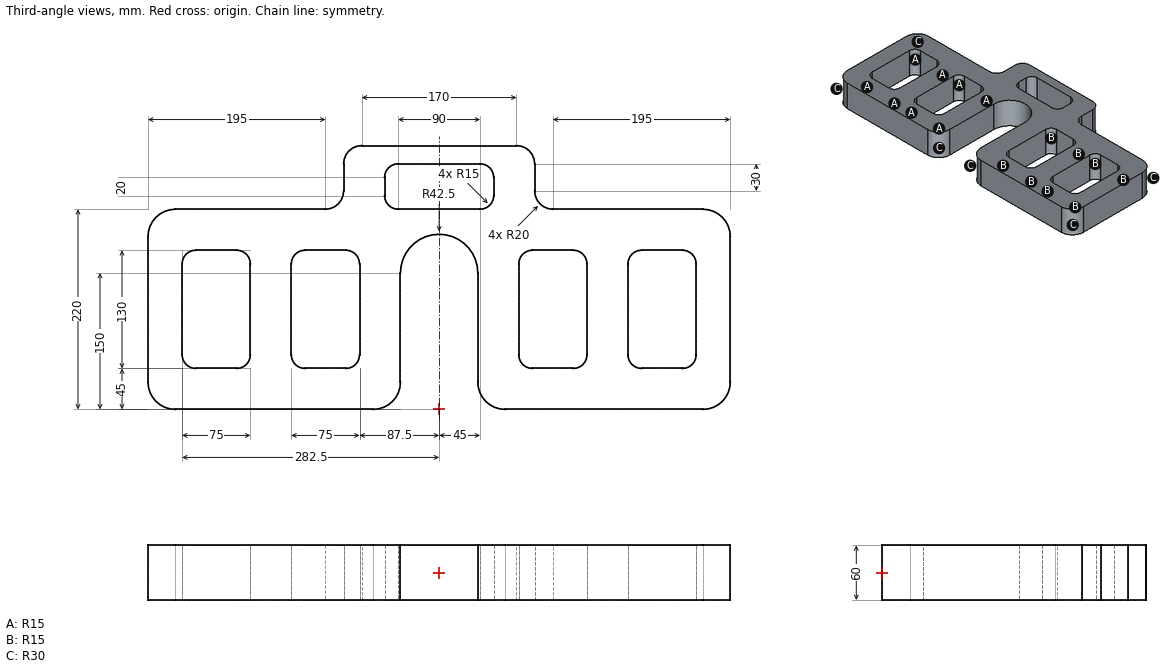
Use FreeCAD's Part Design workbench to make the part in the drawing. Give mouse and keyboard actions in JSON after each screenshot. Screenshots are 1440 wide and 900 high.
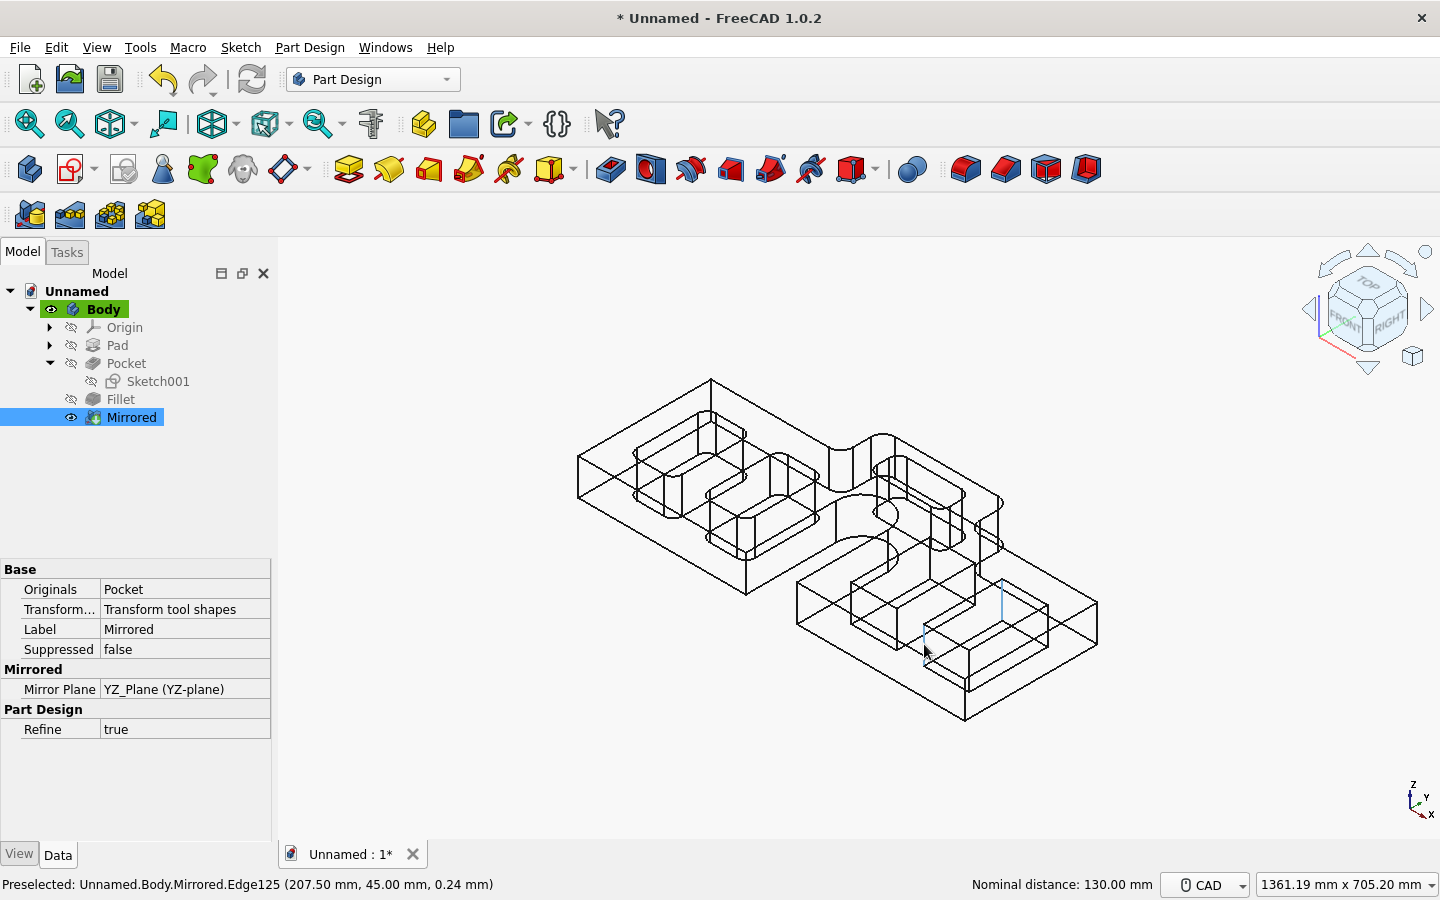
{"action": "left_click", "coordinate": [969, 666], "text": "ctrl"}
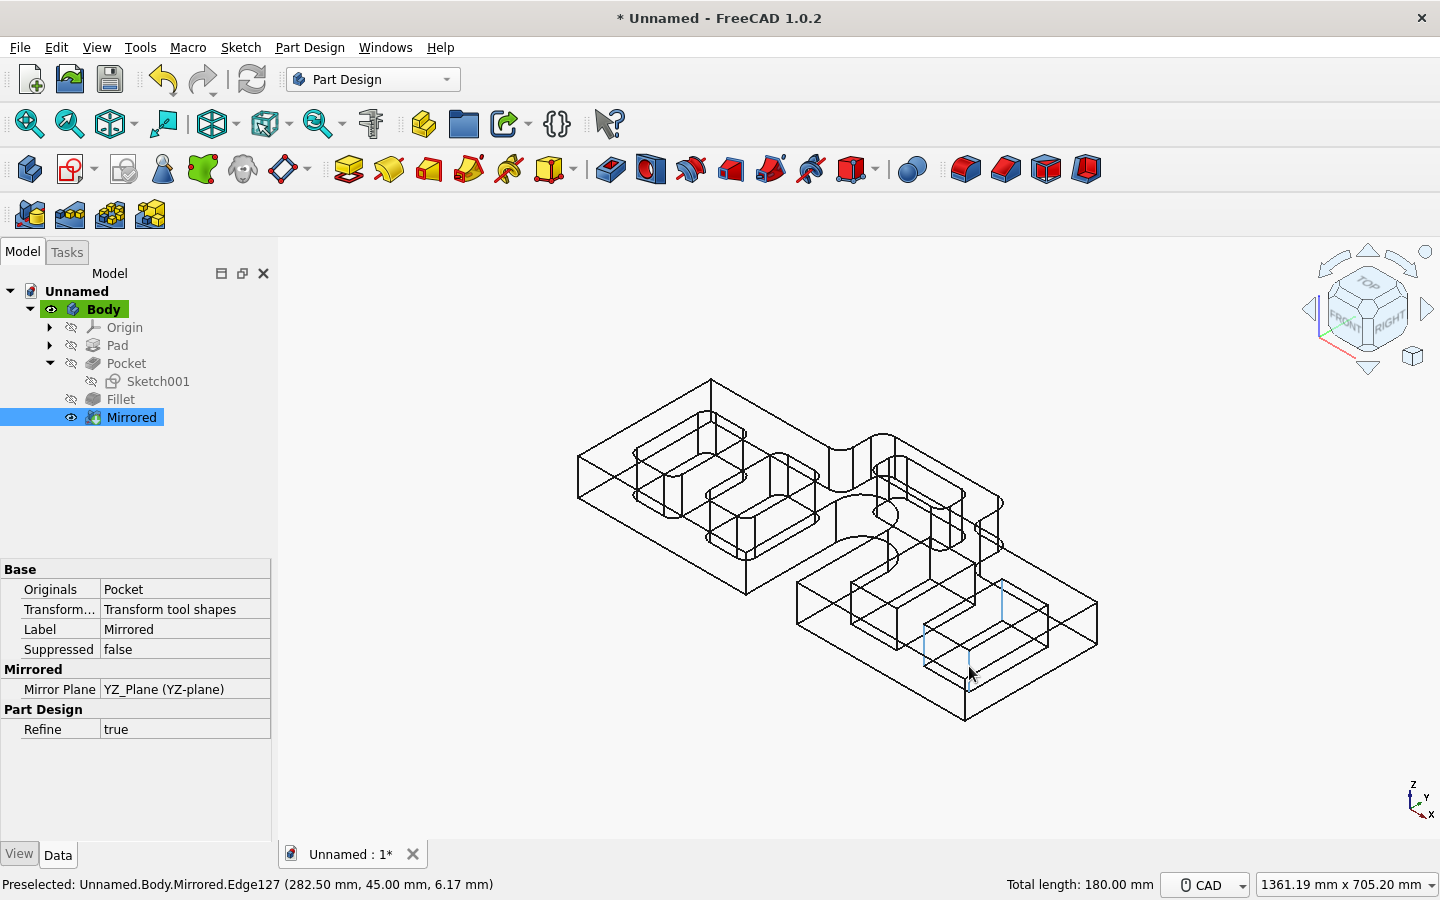
{"action": "left_click", "coordinate": [1048, 621], "text": "ctrl"}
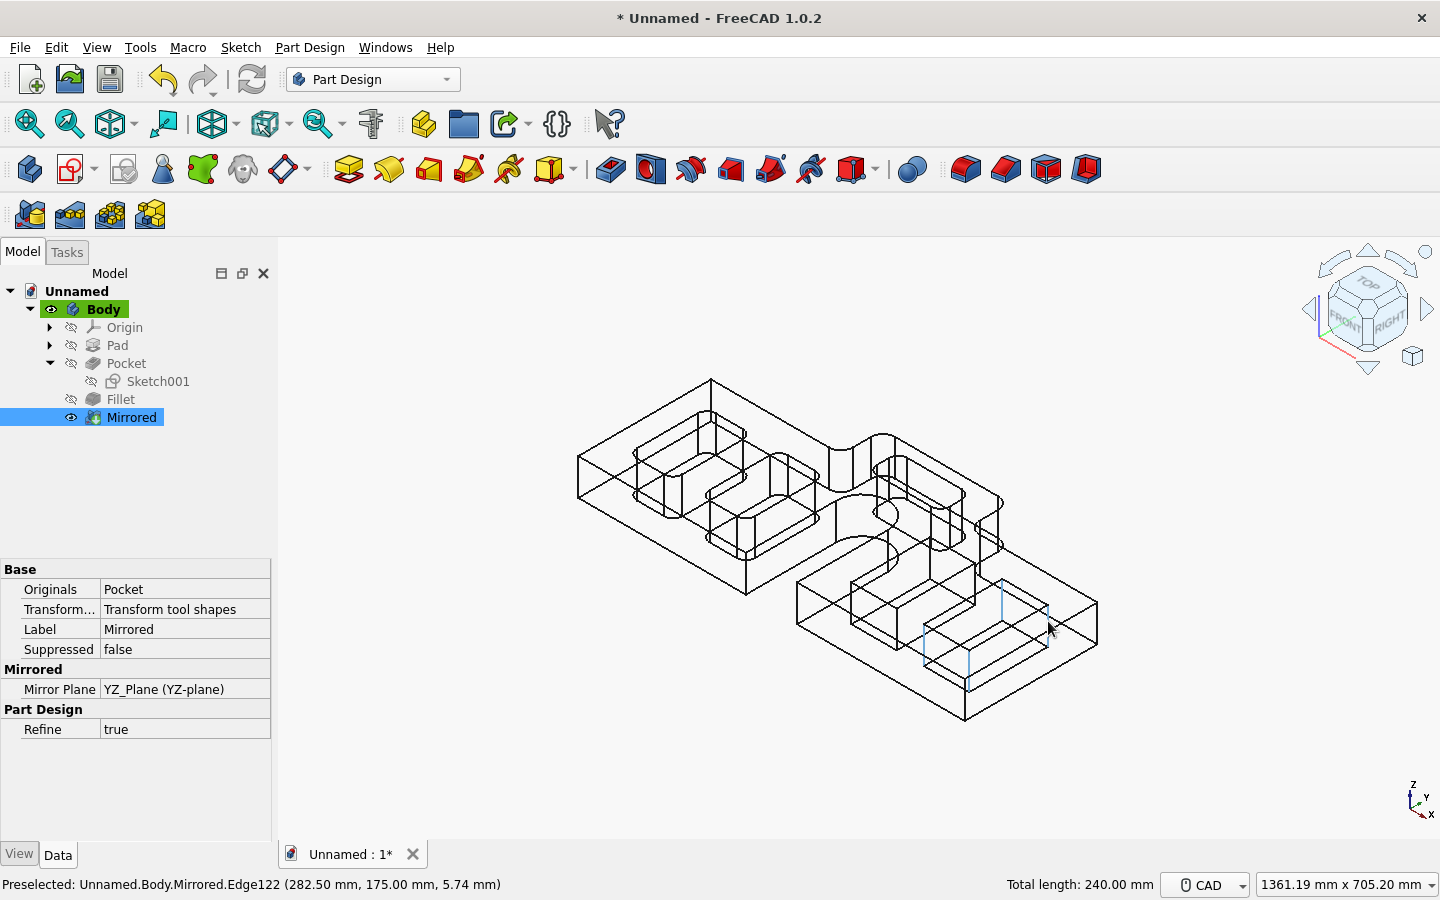
{"action": "left_click", "coordinate": [930, 557], "text": "ctrl"}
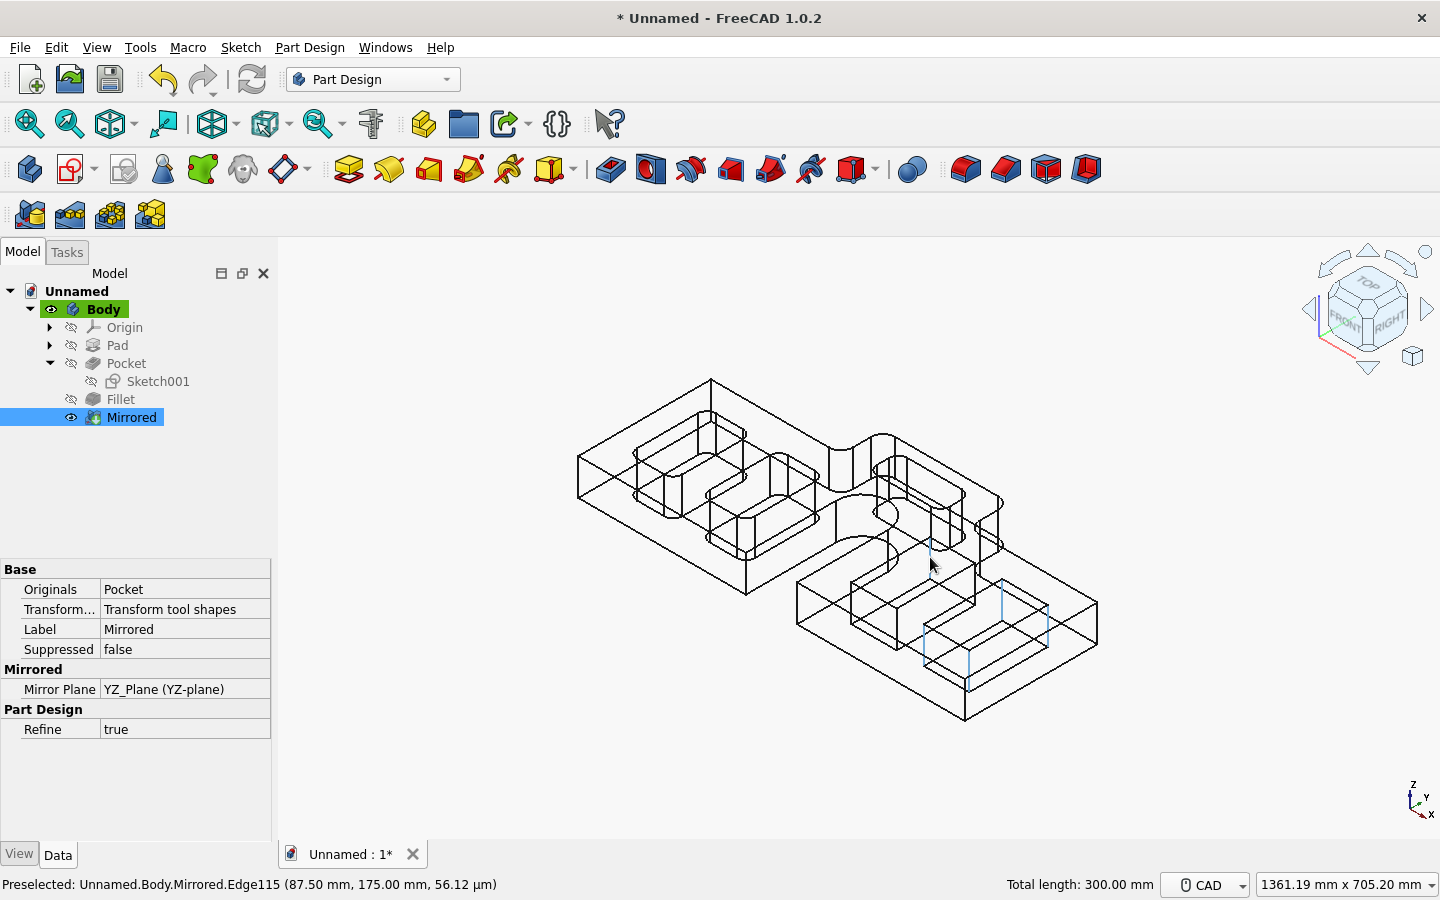
{"action": "left_click", "coordinate": [851, 602], "text": "ctrl"}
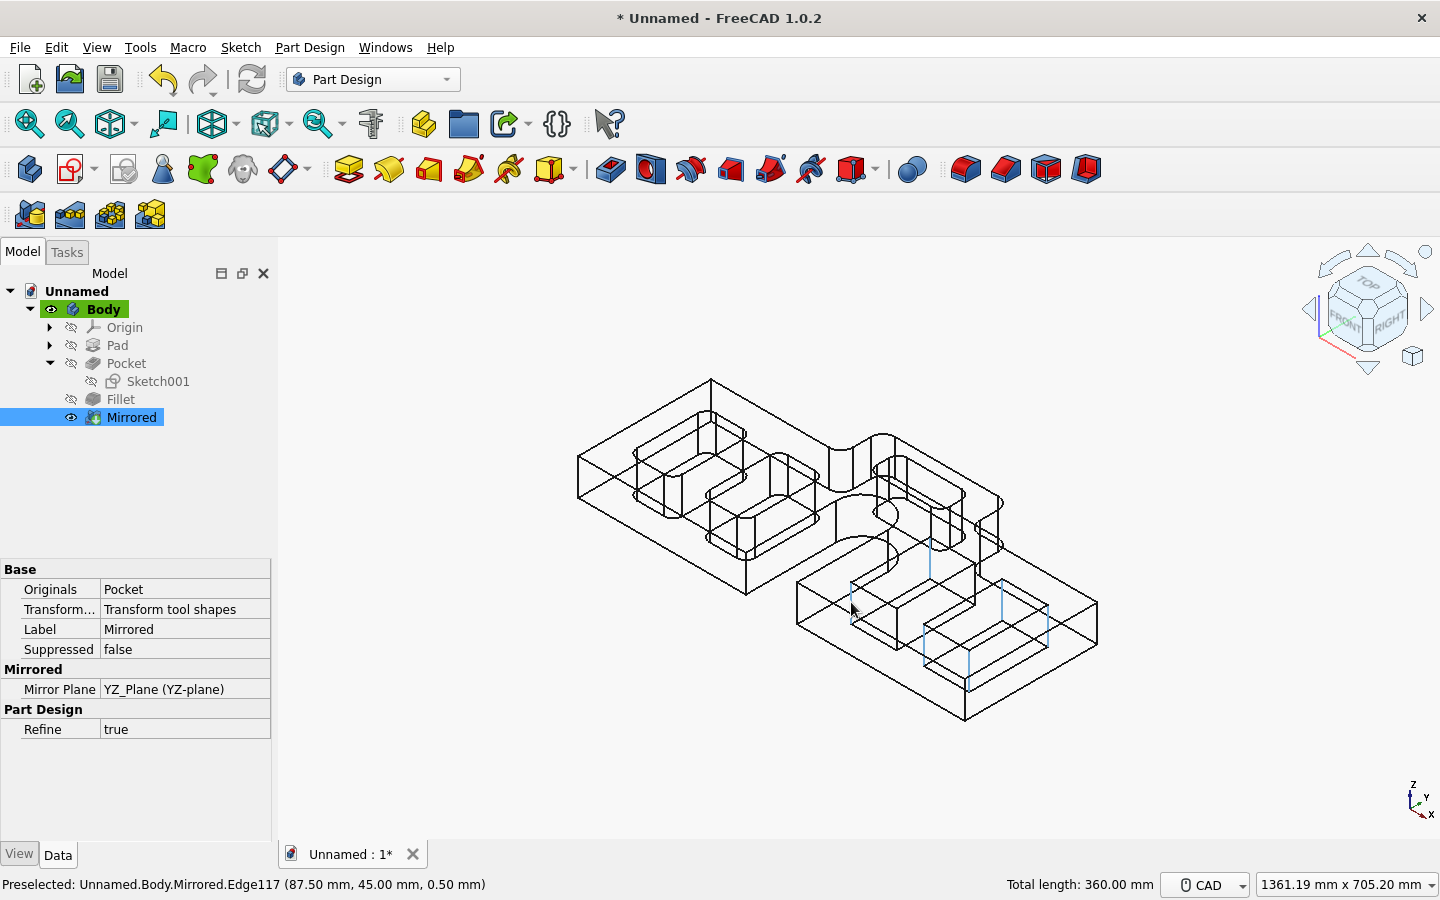
{"action": "left_click", "coordinate": [897, 628], "text": "ctrl"}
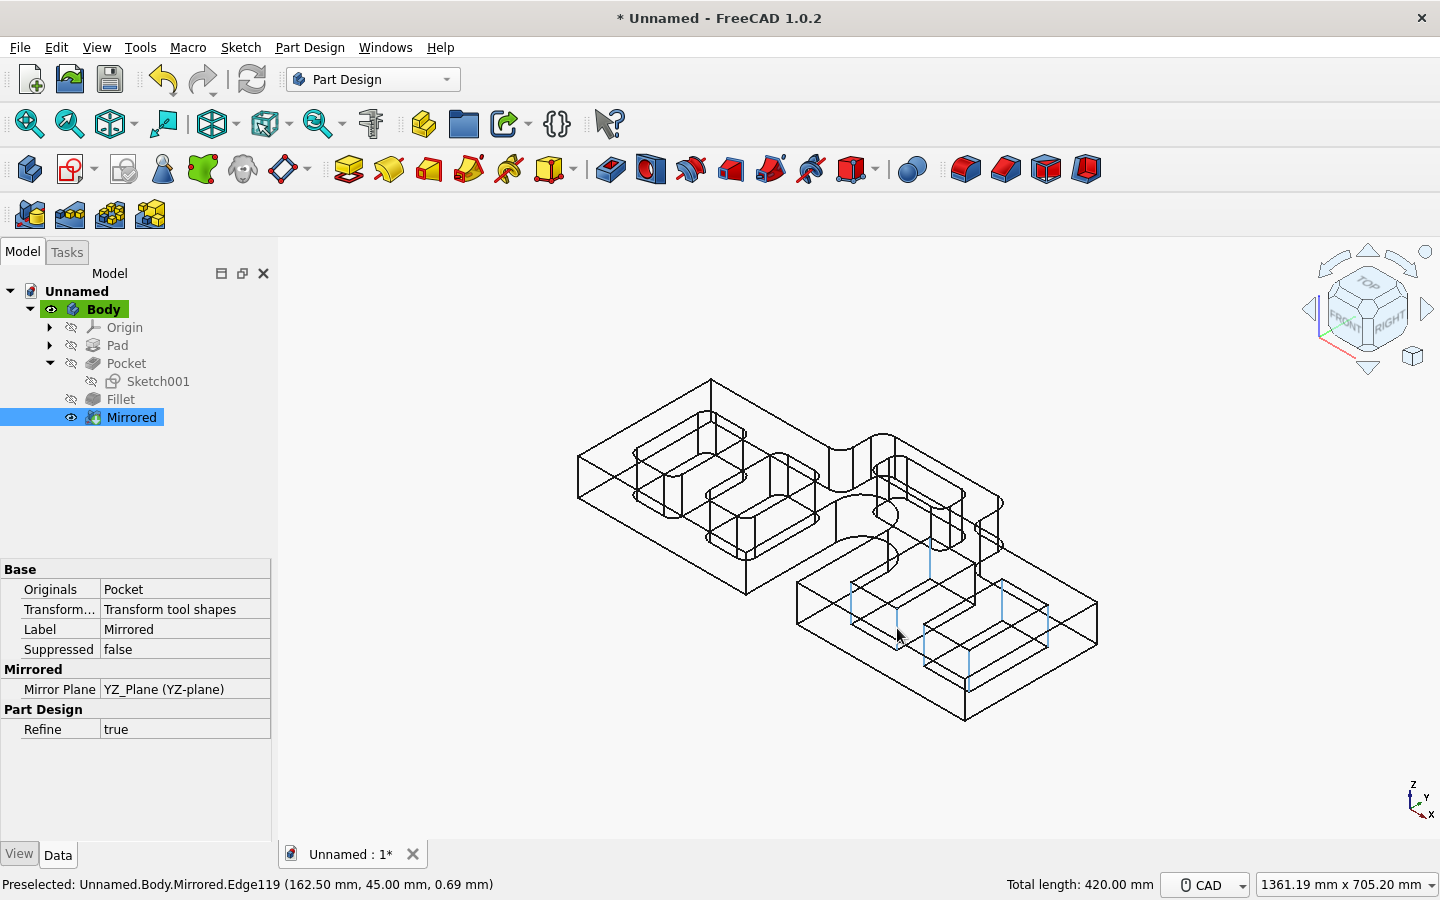
{"action": "left_click", "coordinate": [975, 583], "text": "ctrl"}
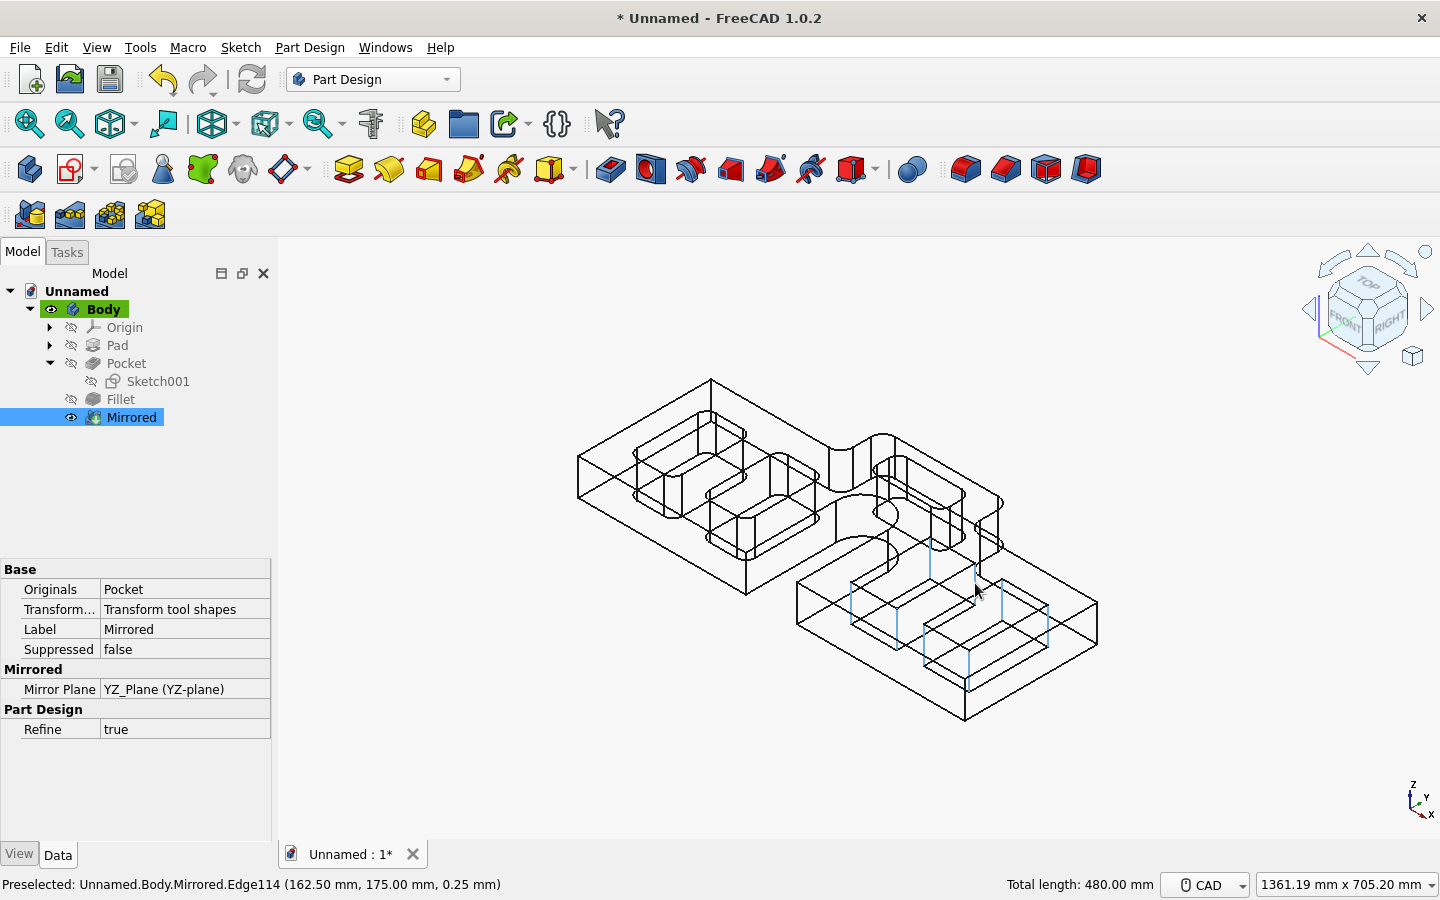
{"action": "key", "text": "v 1"}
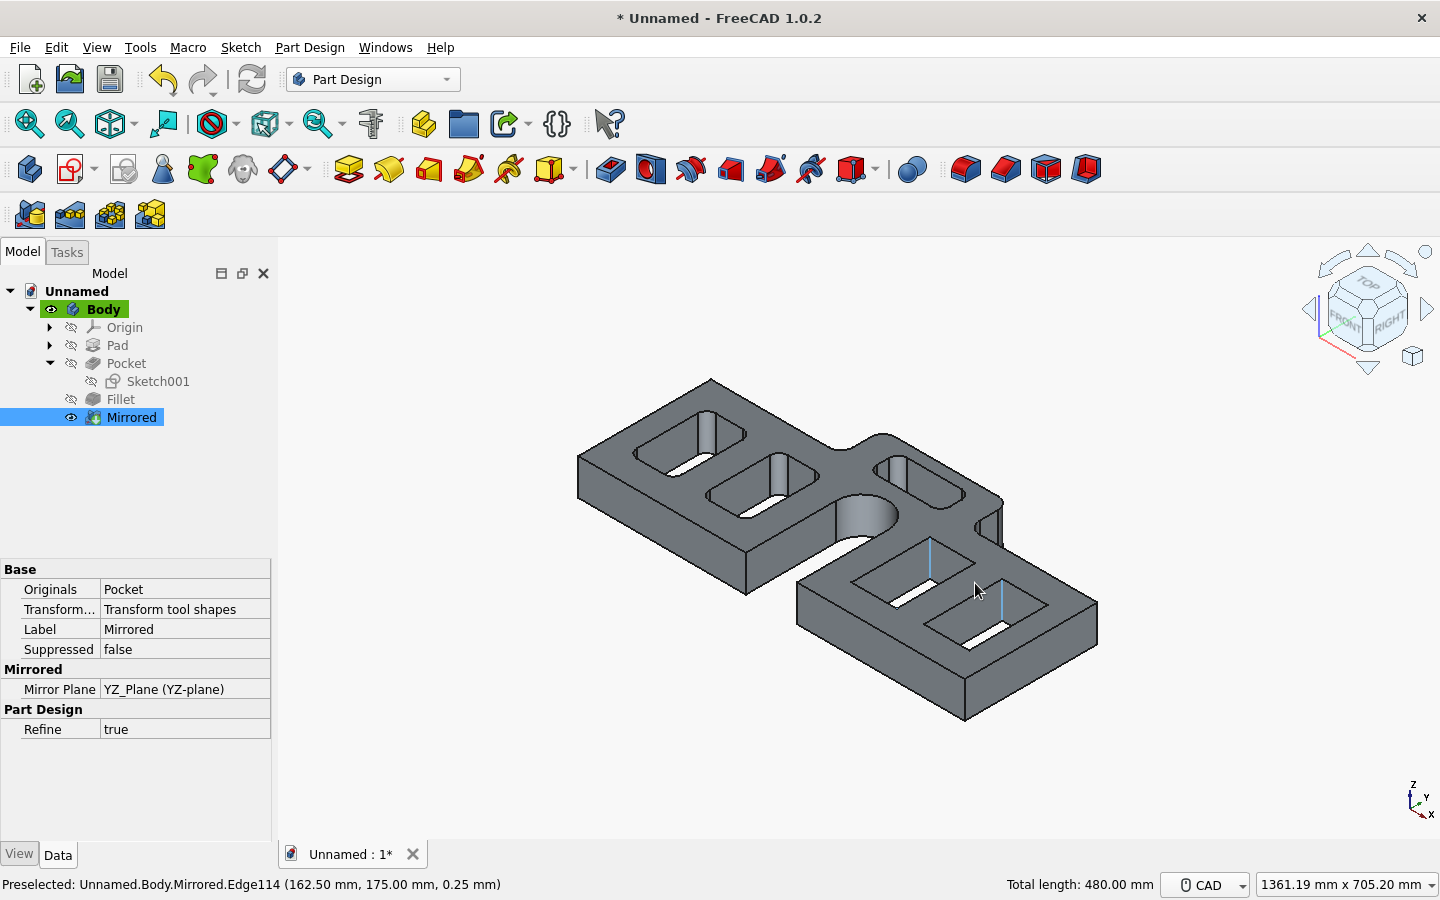
{"action": "left_click", "coordinate": [966, 170]}